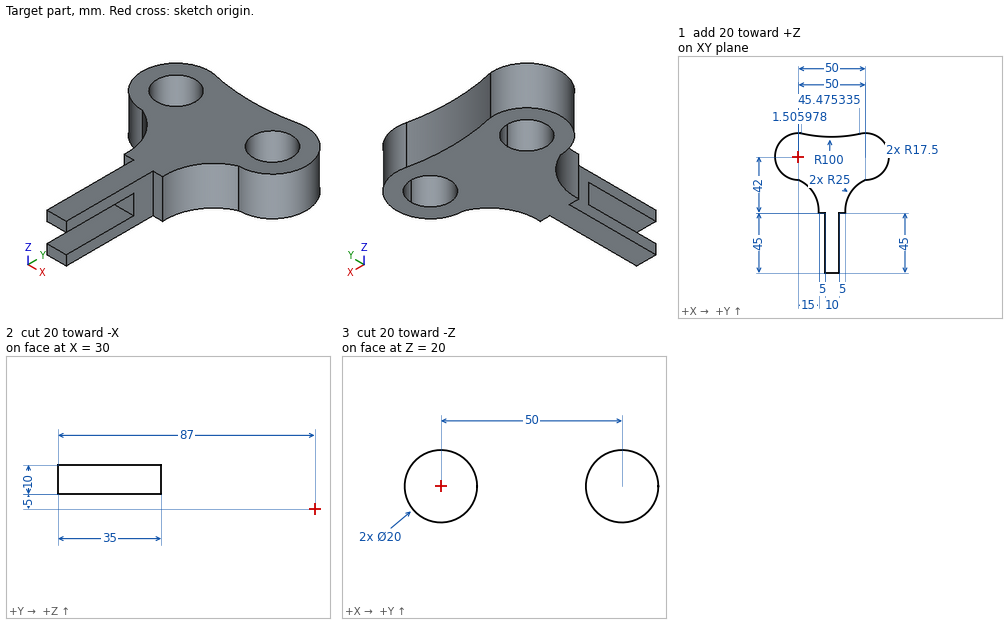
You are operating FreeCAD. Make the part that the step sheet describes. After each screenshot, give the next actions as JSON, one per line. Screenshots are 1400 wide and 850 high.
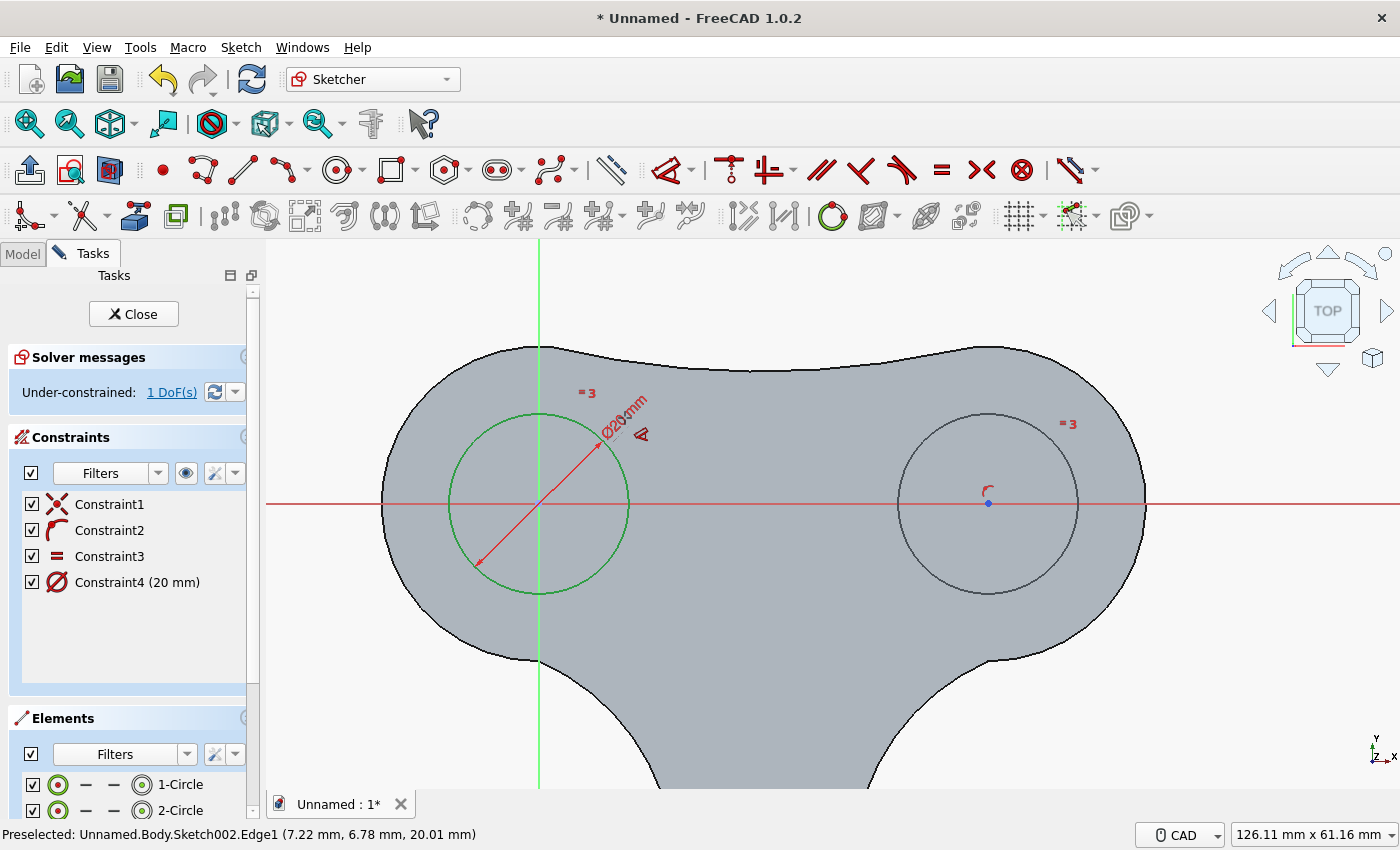
{"action": "left_click", "coordinate": [988, 504]}
{"action": "left_click", "coordinate": [763, 538]}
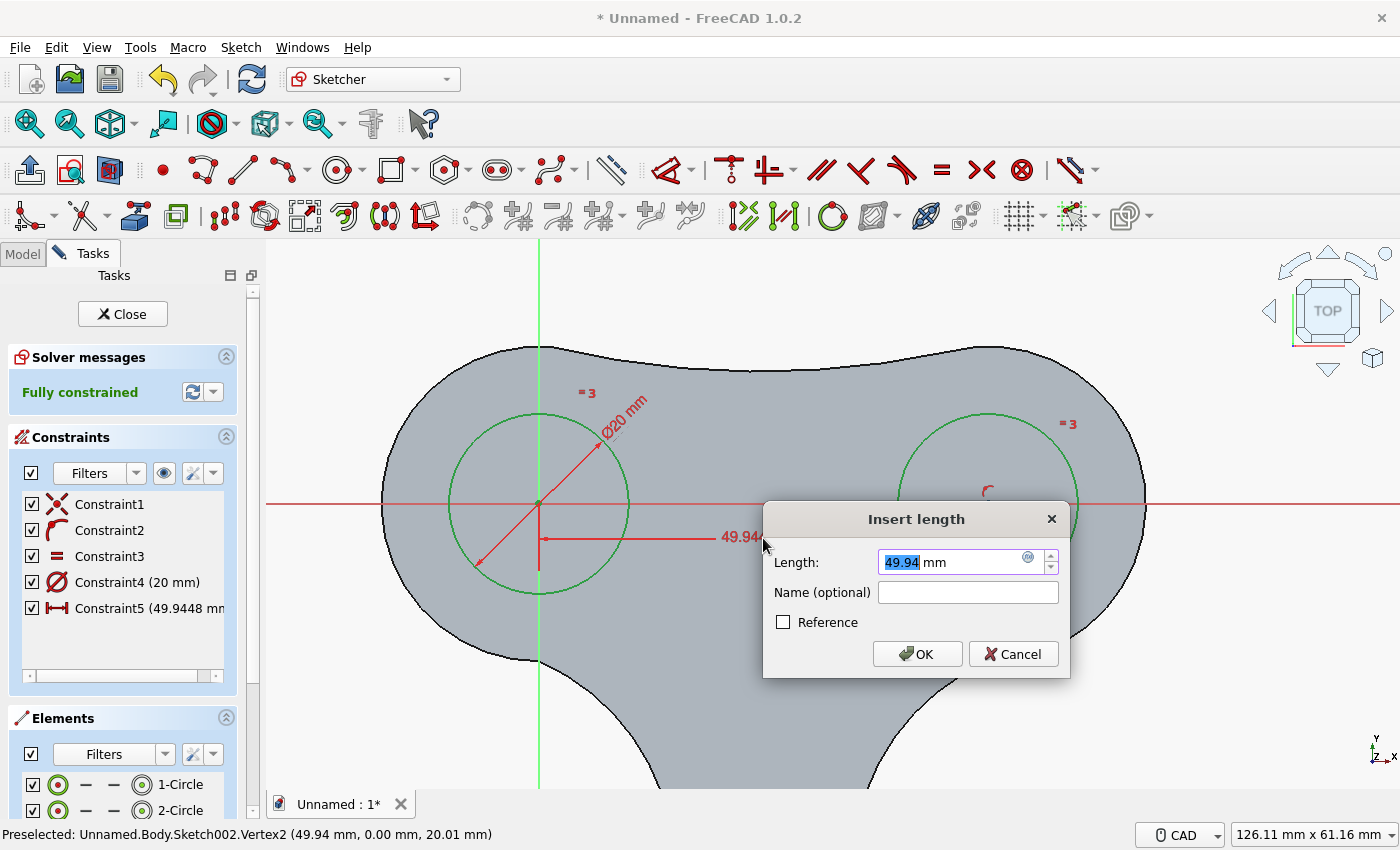
{"action": "type", "text": "50"}
{"action": "key", "text": "Return"}
{"action": "key", "text": "Escape"}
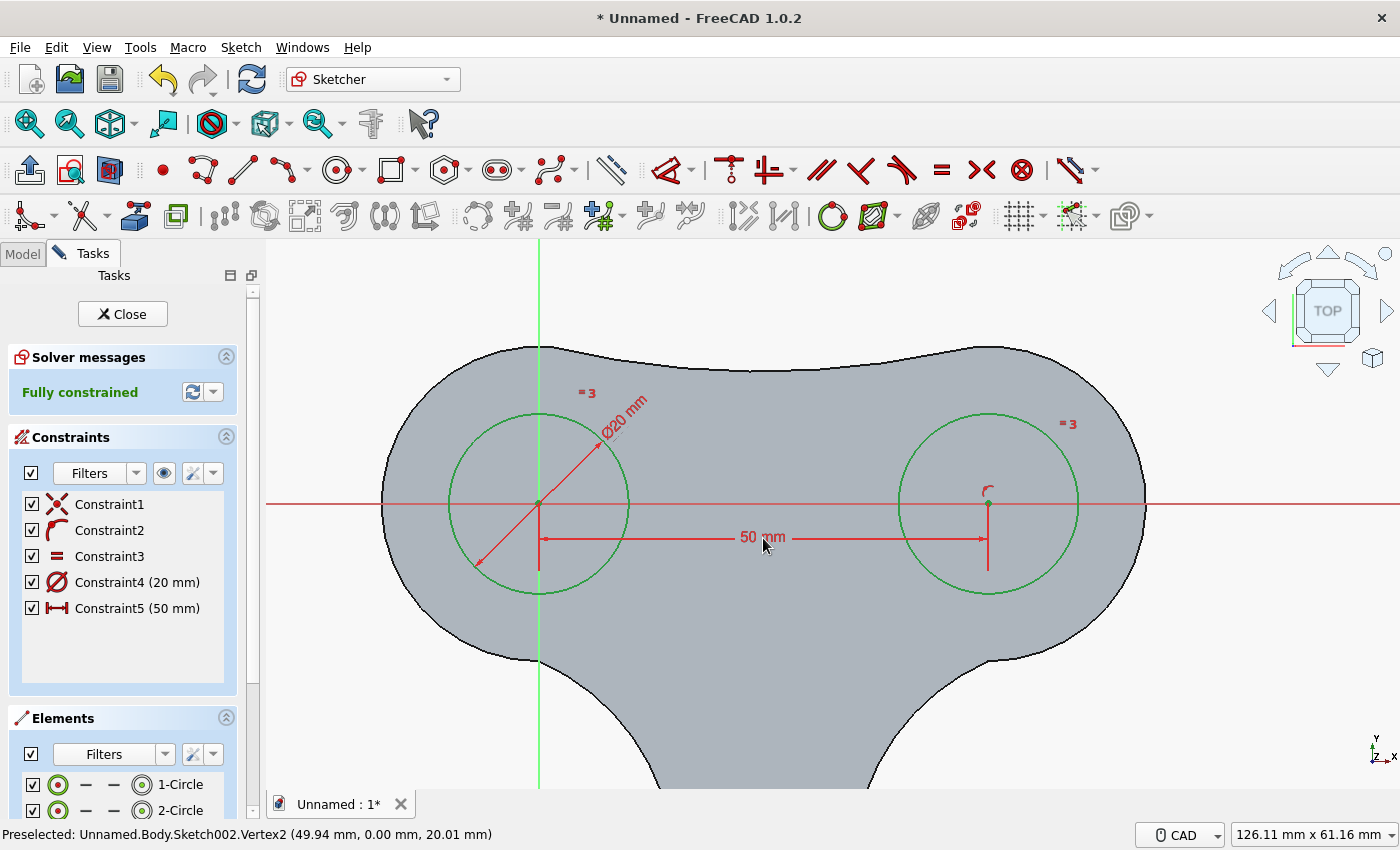
{"action": "left_click", "coordinate": [123, 314]}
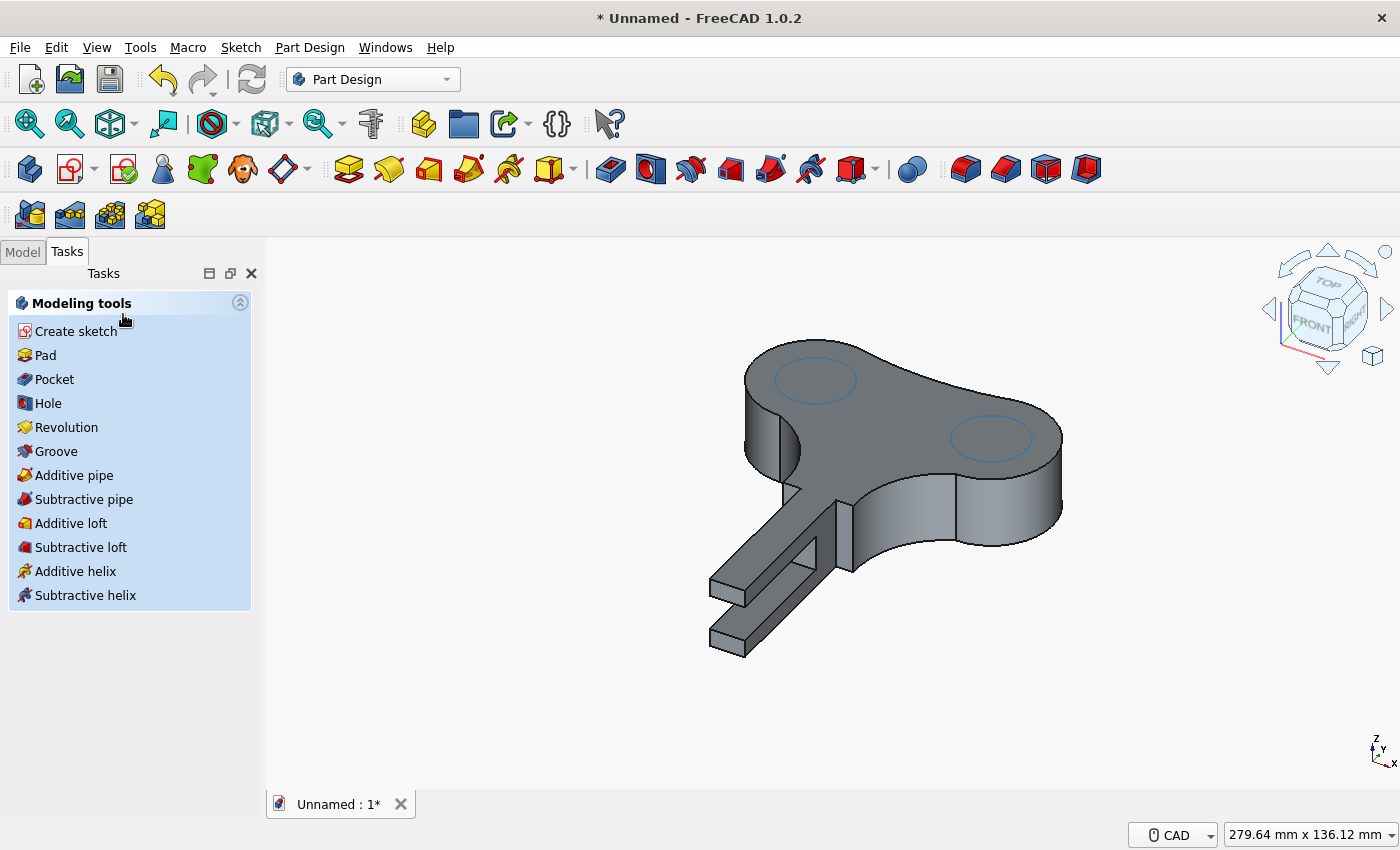
{"action": "left_click", "coordinate": [612, 170]}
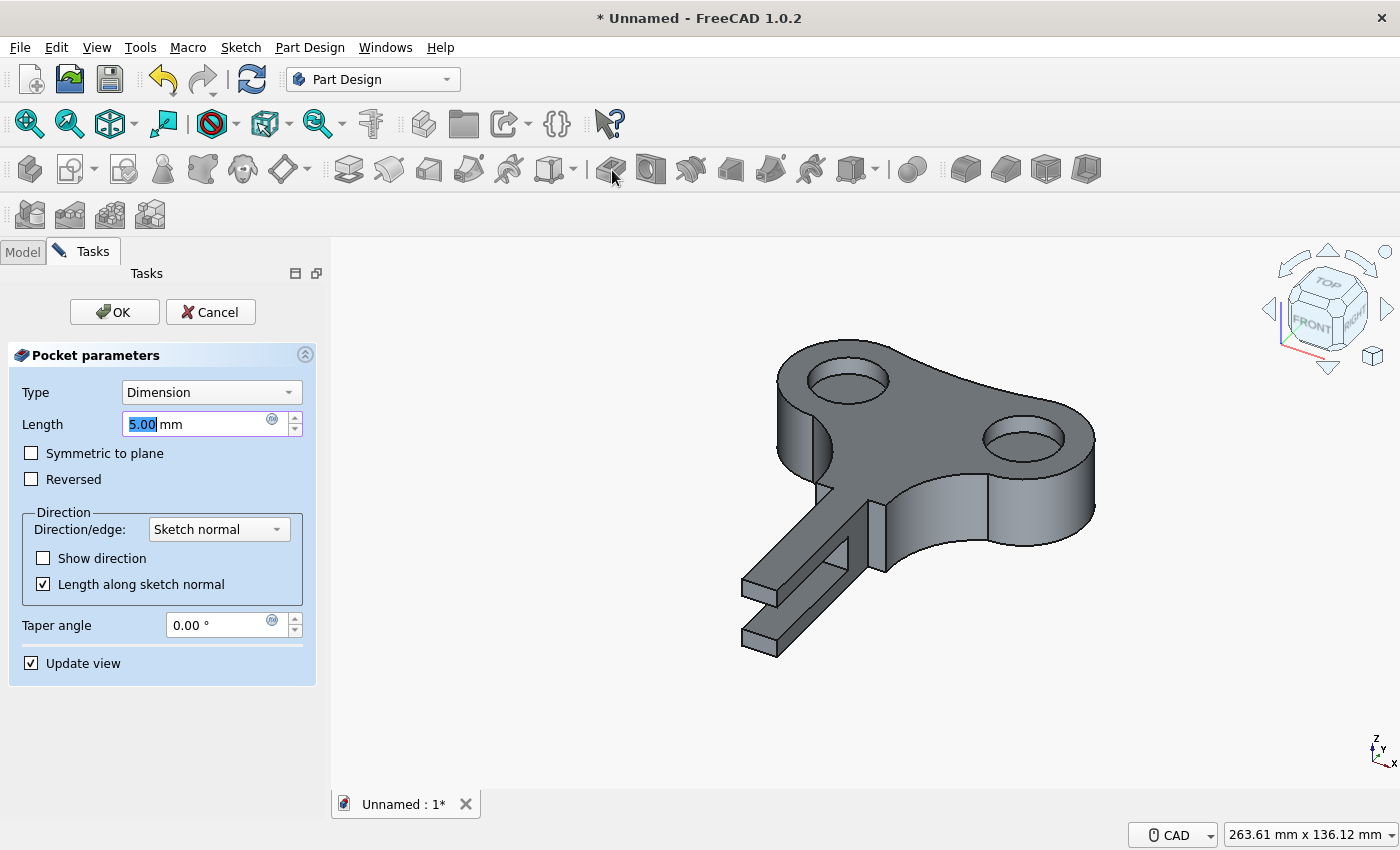
{"action": "type", "text": "20"}
{"action": "key", "text": "Tab"}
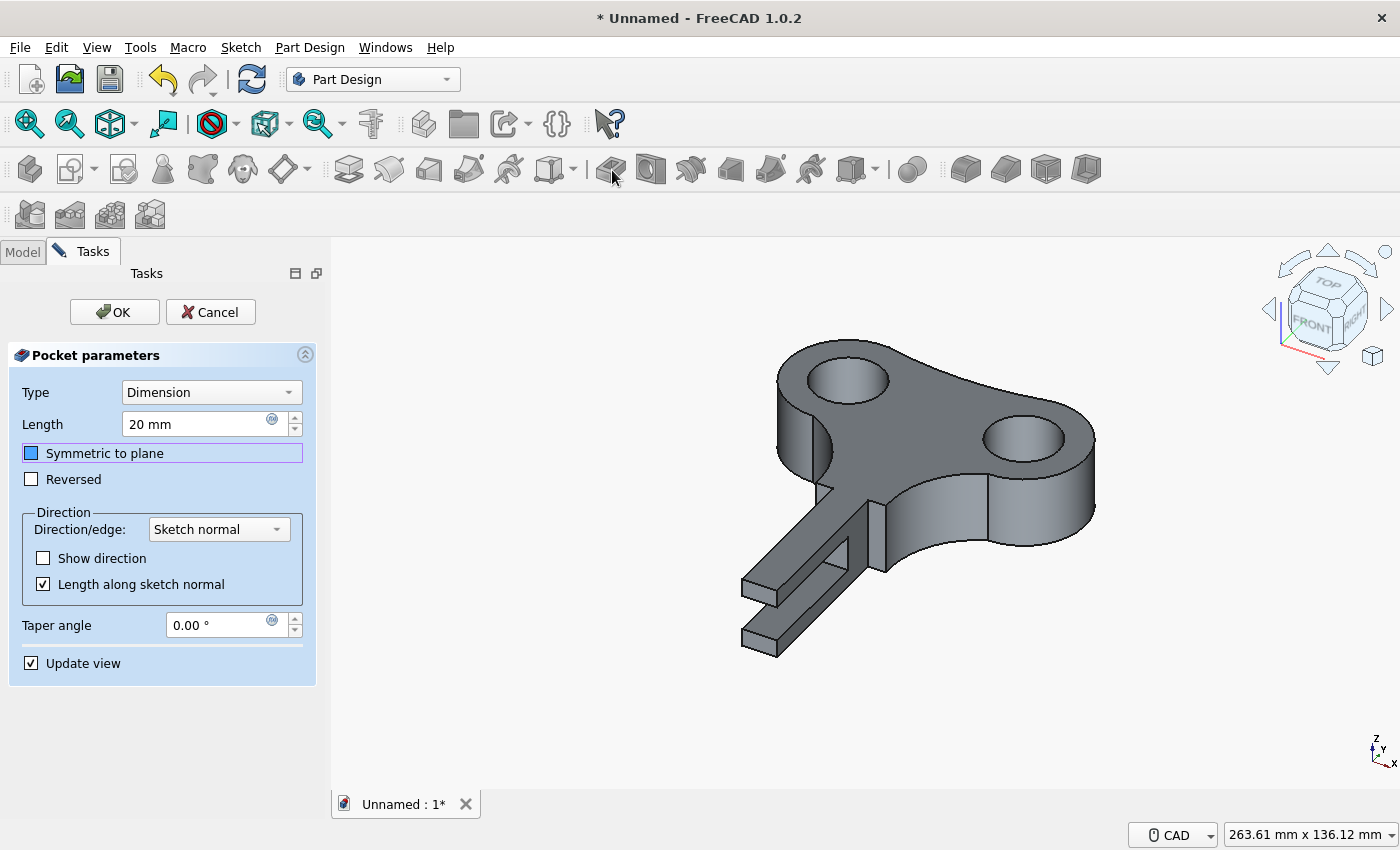
{"action": "left_click", "coordinate": [115, 312]}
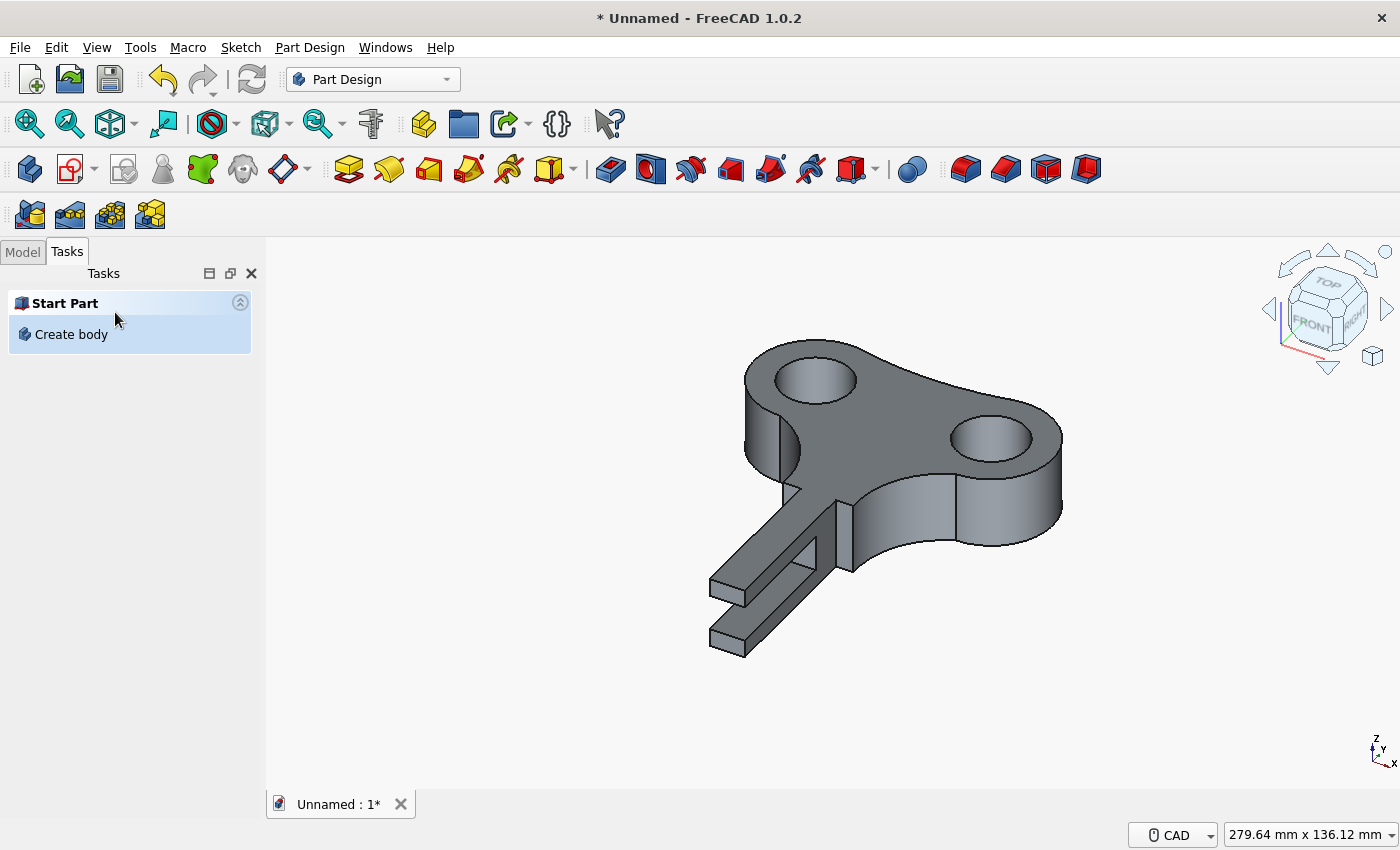
{"action": "key", "text": "0"}